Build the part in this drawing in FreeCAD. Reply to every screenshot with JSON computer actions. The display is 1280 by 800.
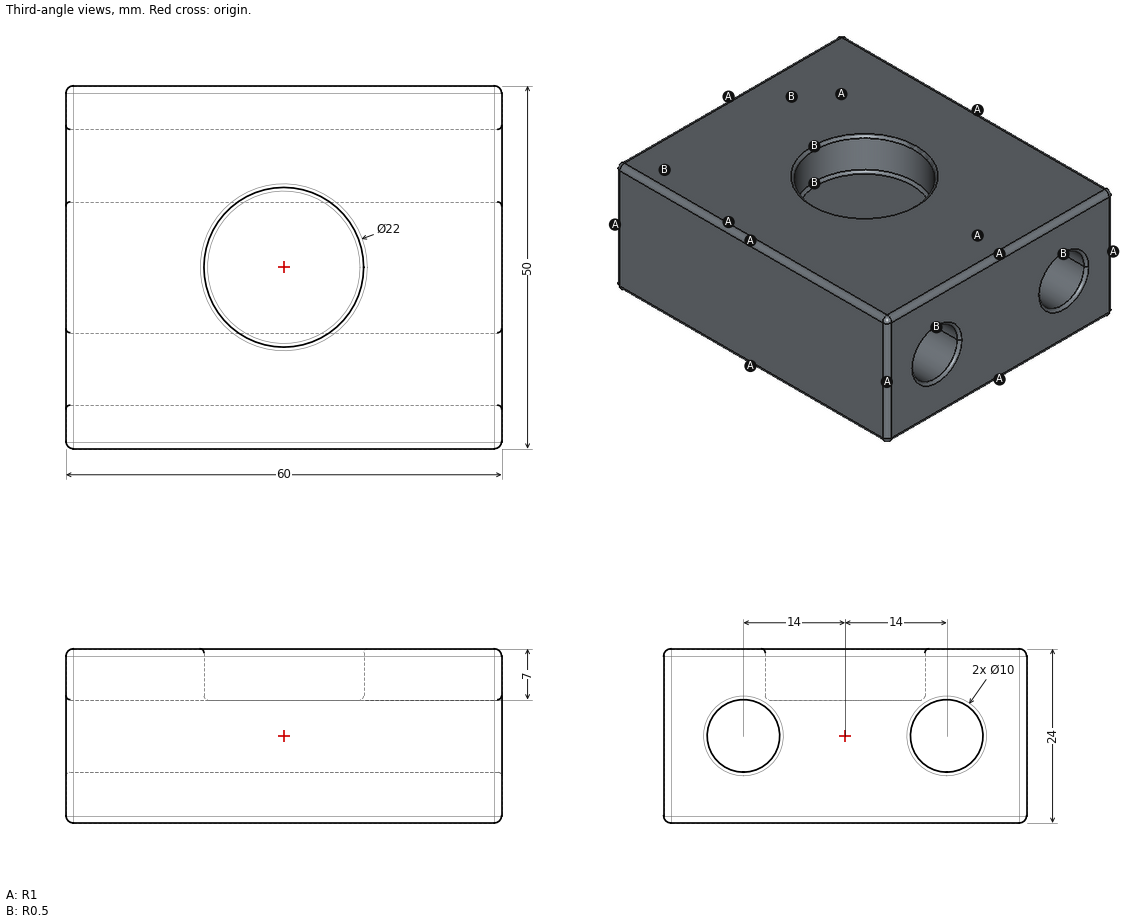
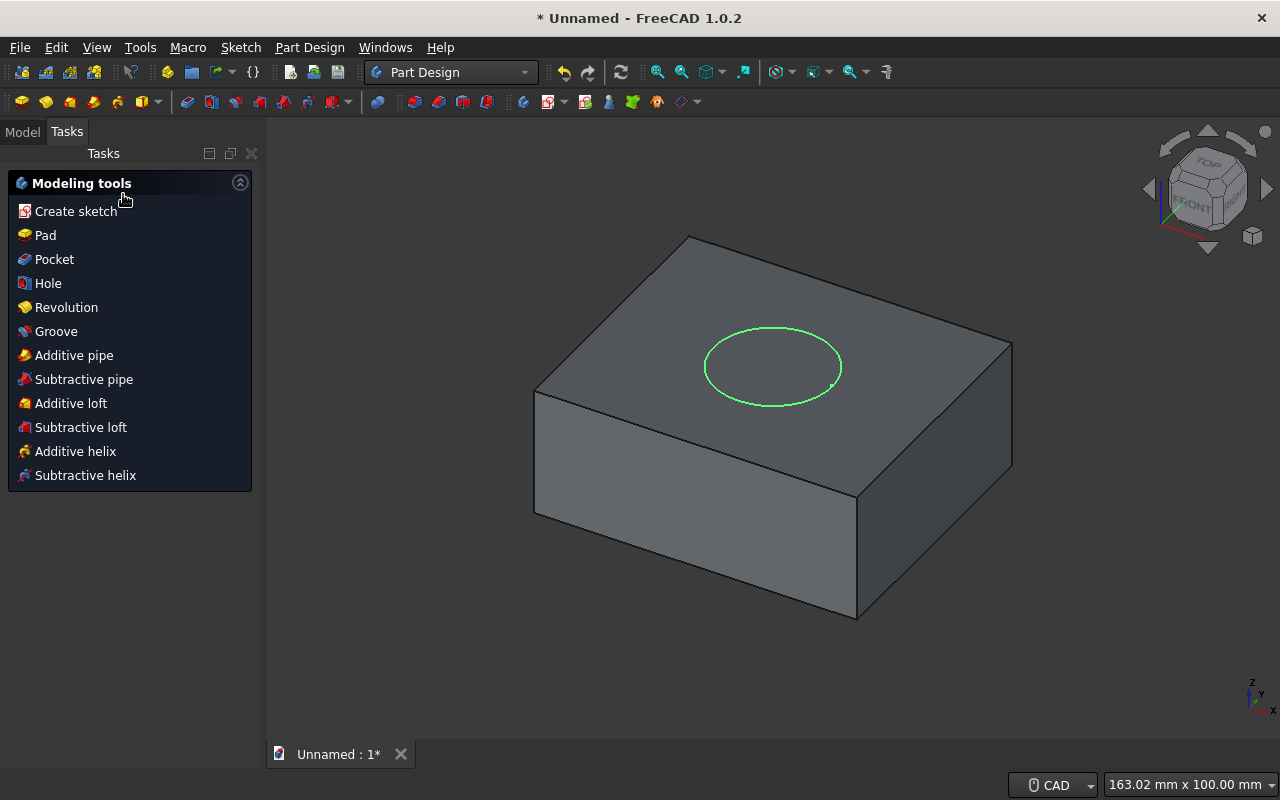
{"action": "left_click", "coordinate": [188, 102]}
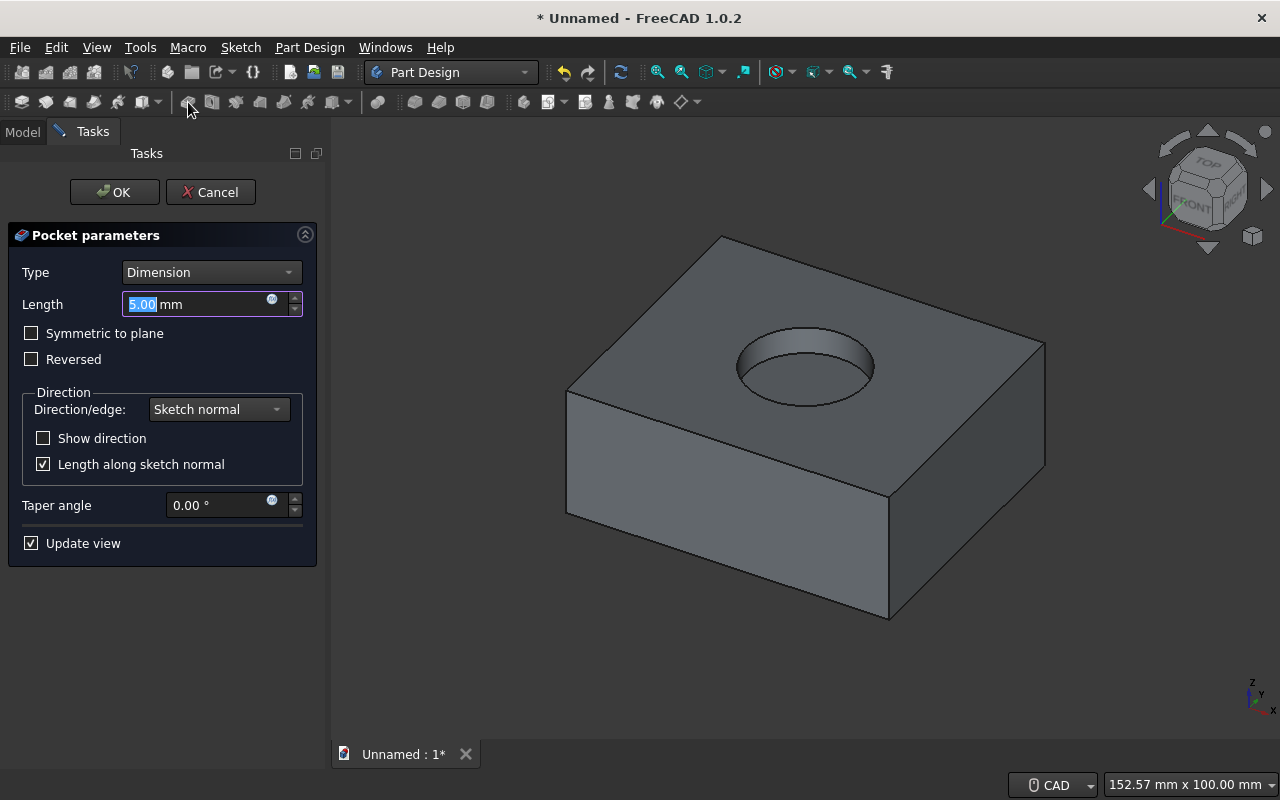
{"action": "type", "text": "7"}
{"action": "key", "text": "Tab"}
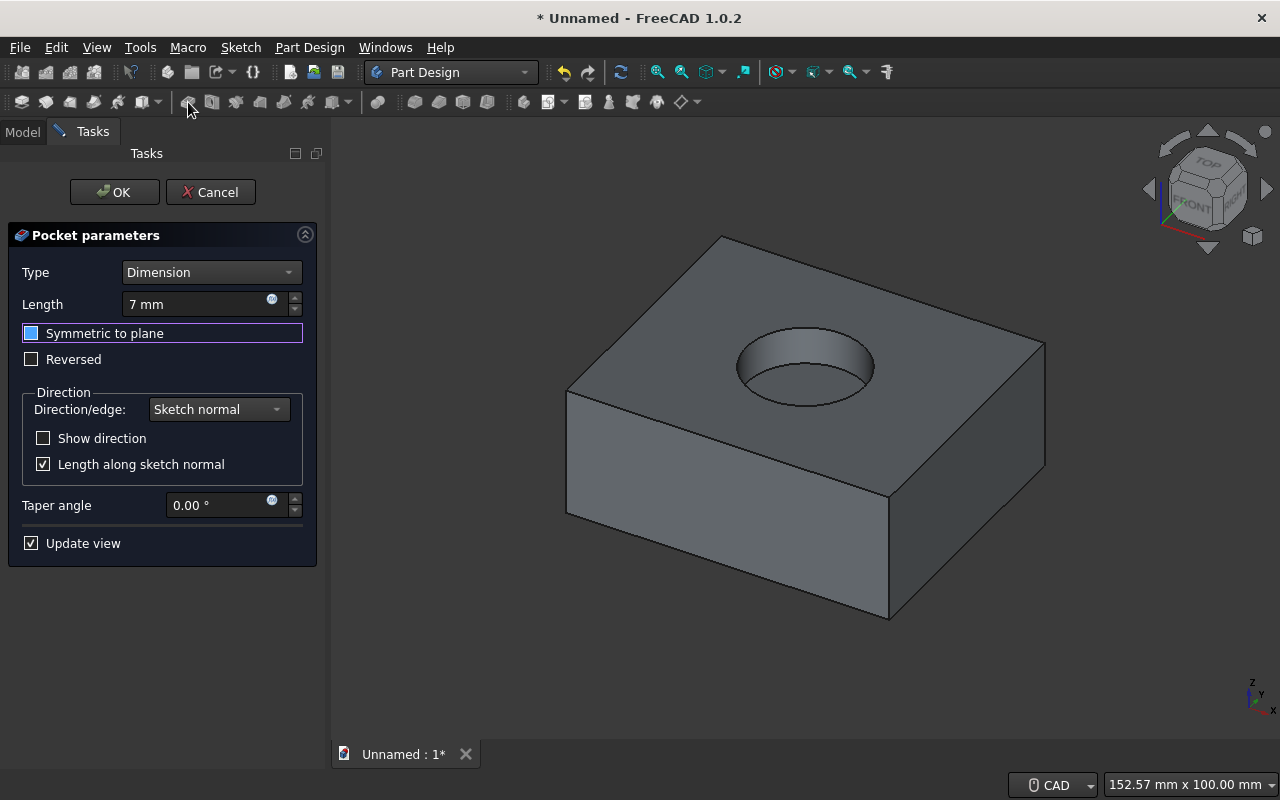
{"action": "left_click", "coordinate": [115, 192]}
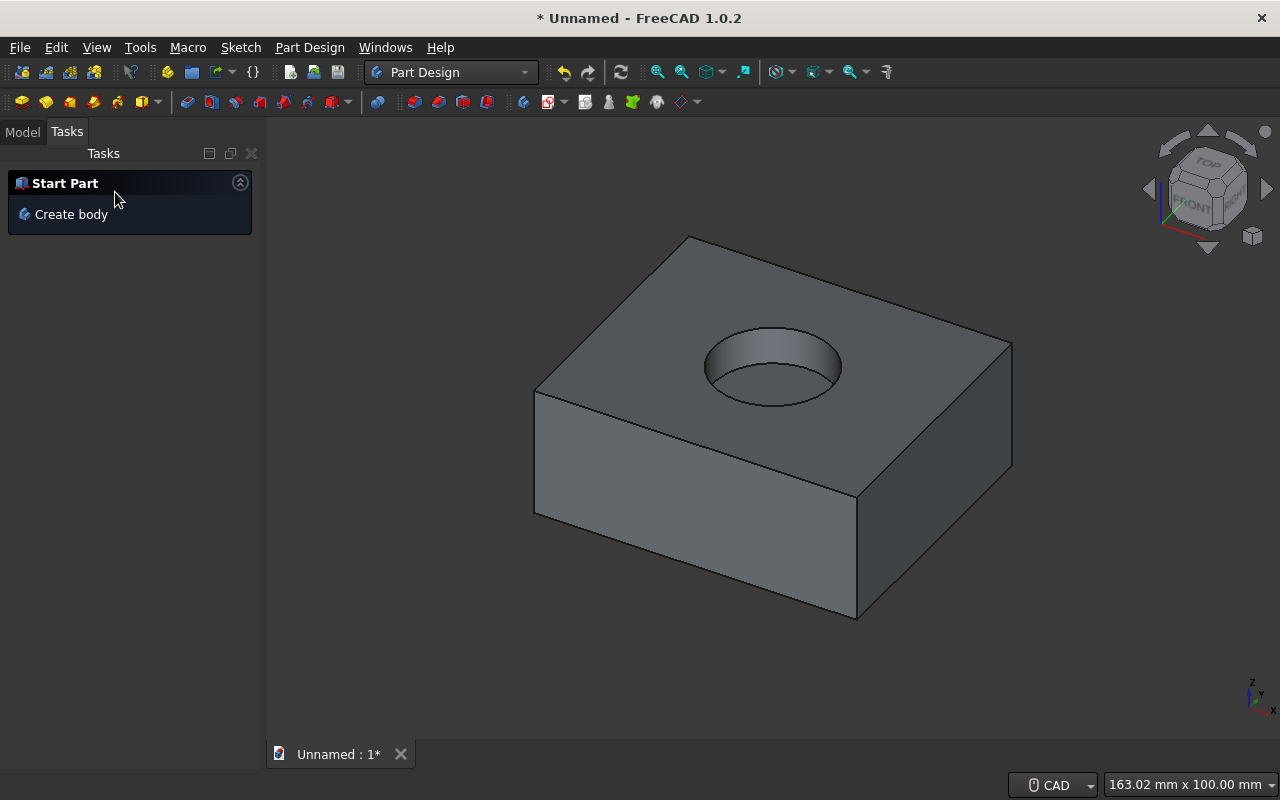
{"action": "left_click", "coordinate": [957, 458]}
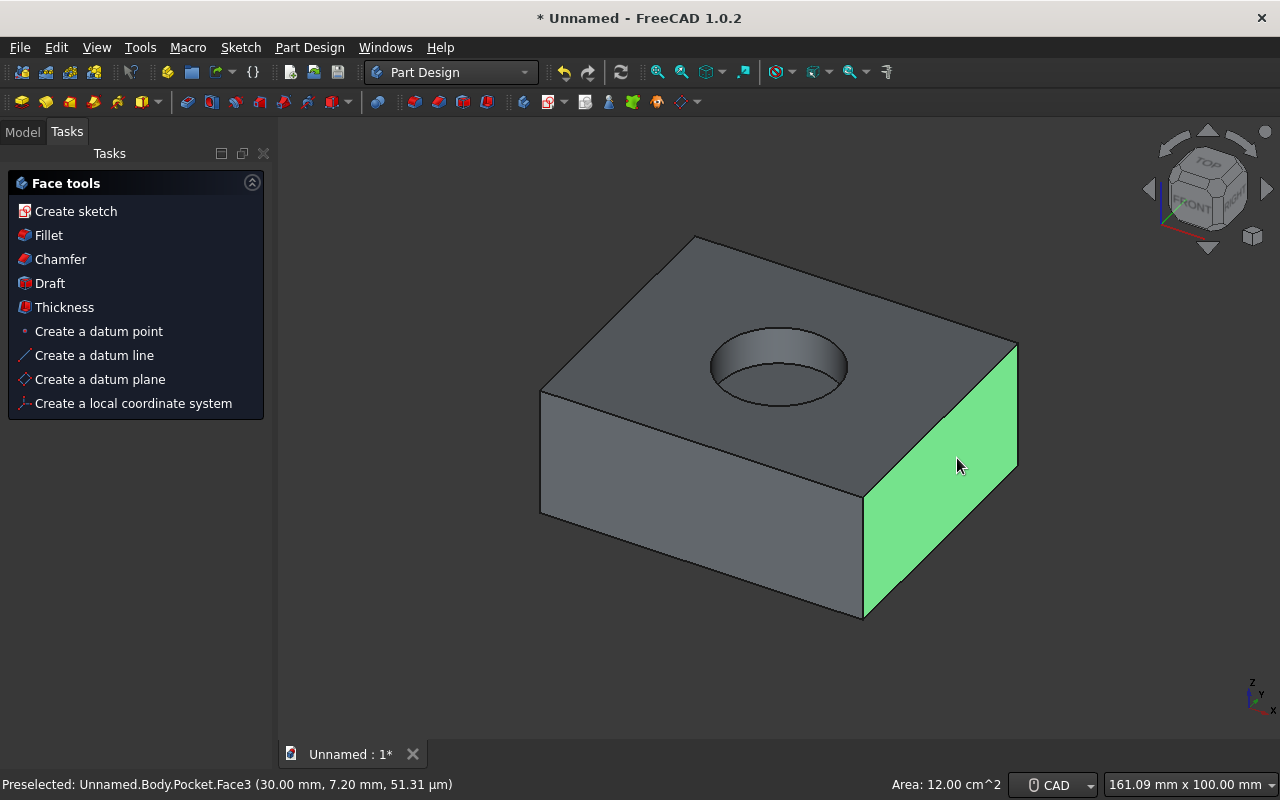
{"action": "left_click", "coordinate": [548, 102]}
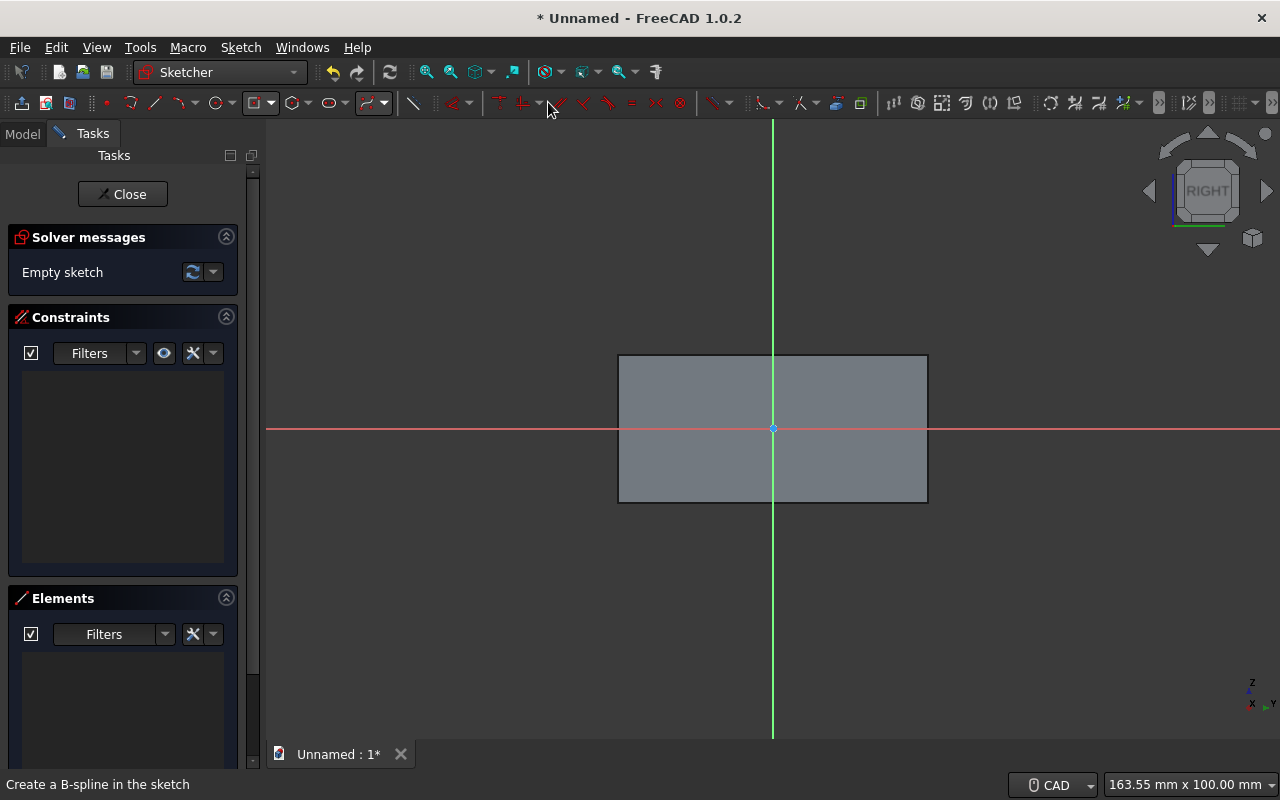
{"action": "scroll", "coordinate": [829, 429], "scroll_direction": "up", "scroll_amount": 4}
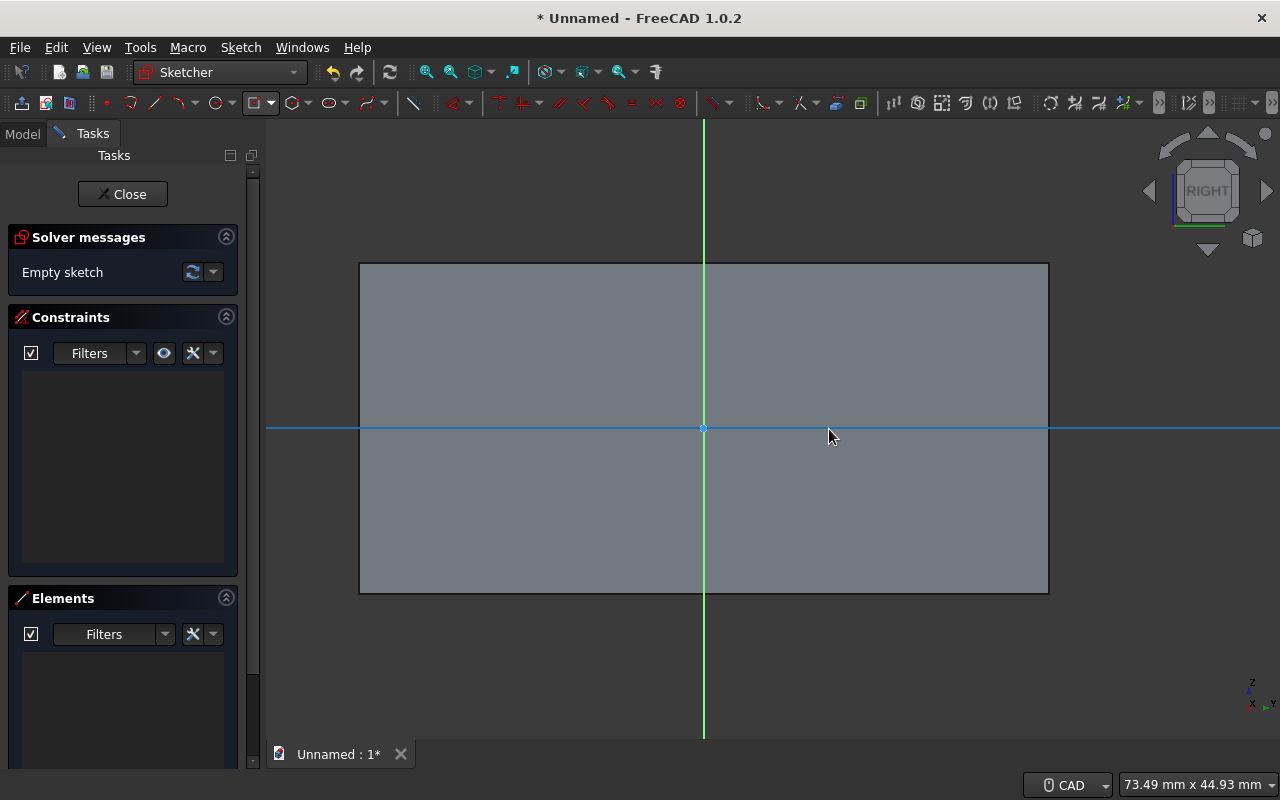
{"action": "left_click", "coordinate": [216, 104]}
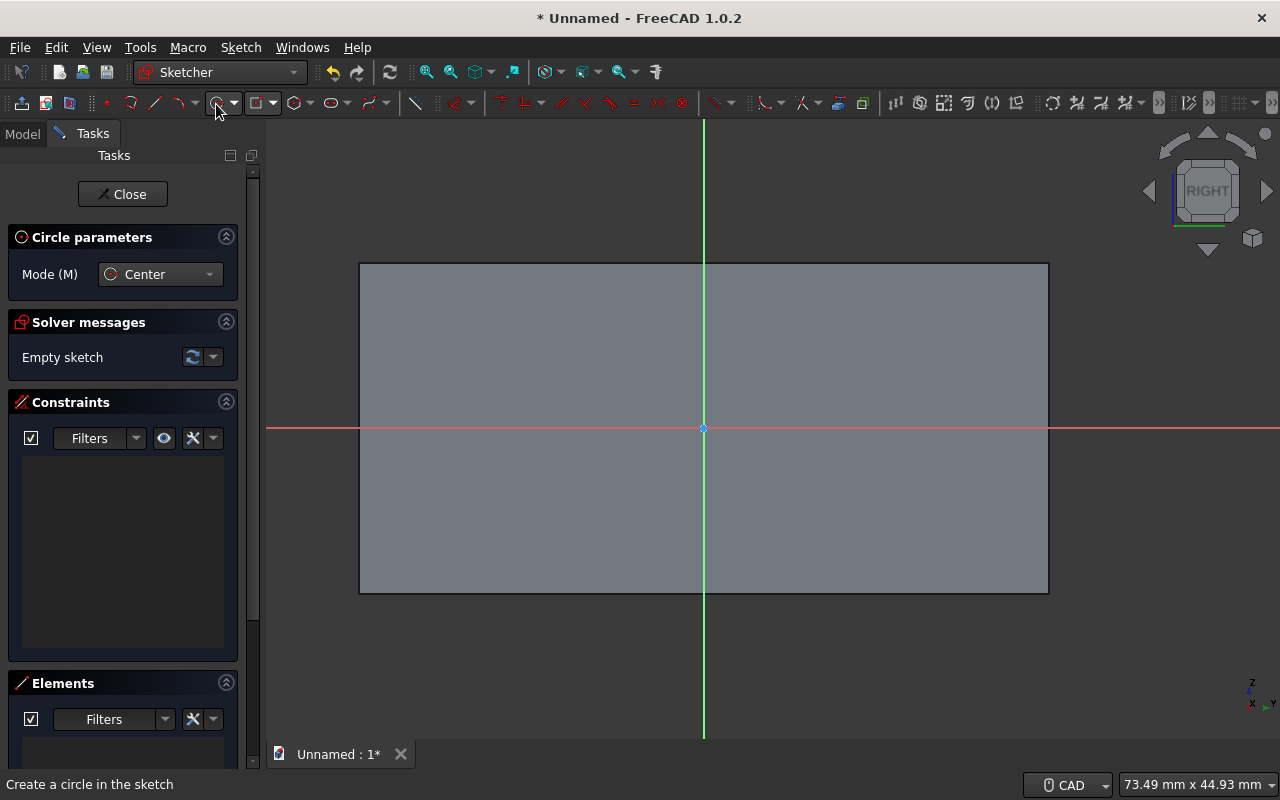
{"action": "left_click", "coordinate": [897, 428]}
{"action": "mouse_move", "coordinate": [946, 380]}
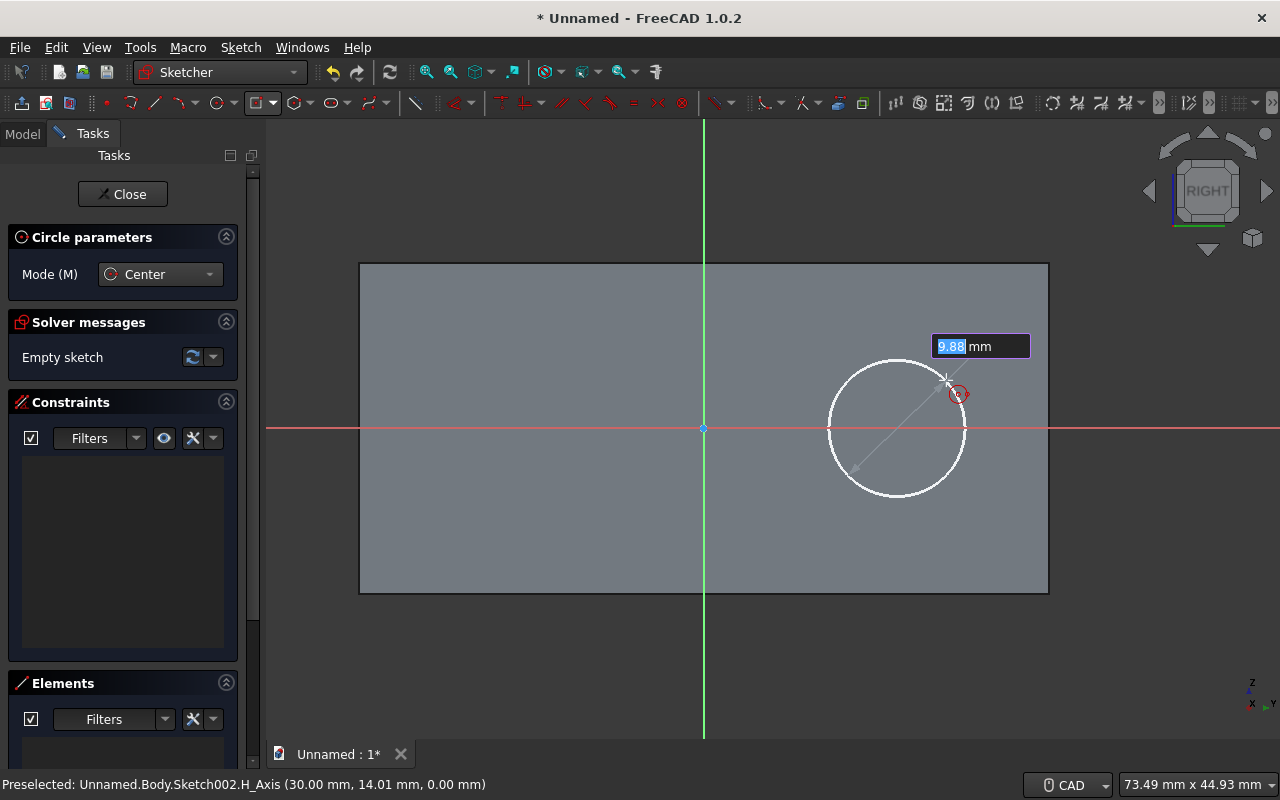
{"action": "type", "text": "10"}
{"action": "key", "text": "Return"}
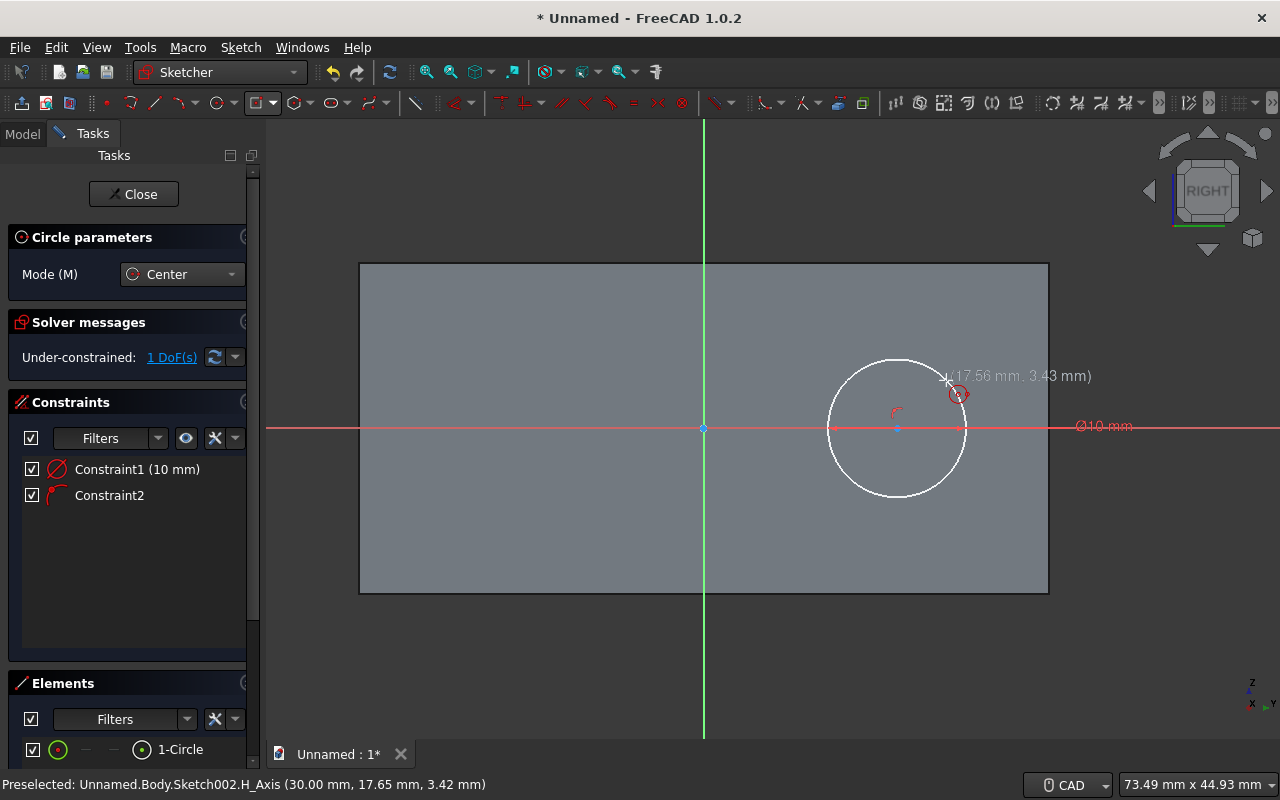
{"action": "left_click", "coordinate": [511, 428]}
{"action": "mouse_move", "coordinate": [559, 380]}